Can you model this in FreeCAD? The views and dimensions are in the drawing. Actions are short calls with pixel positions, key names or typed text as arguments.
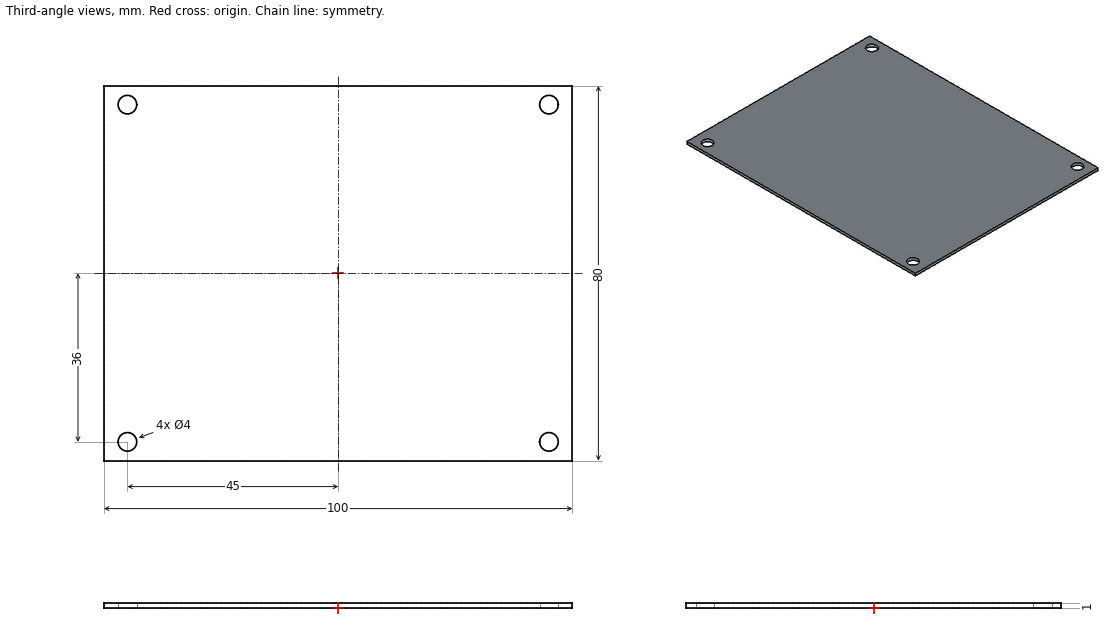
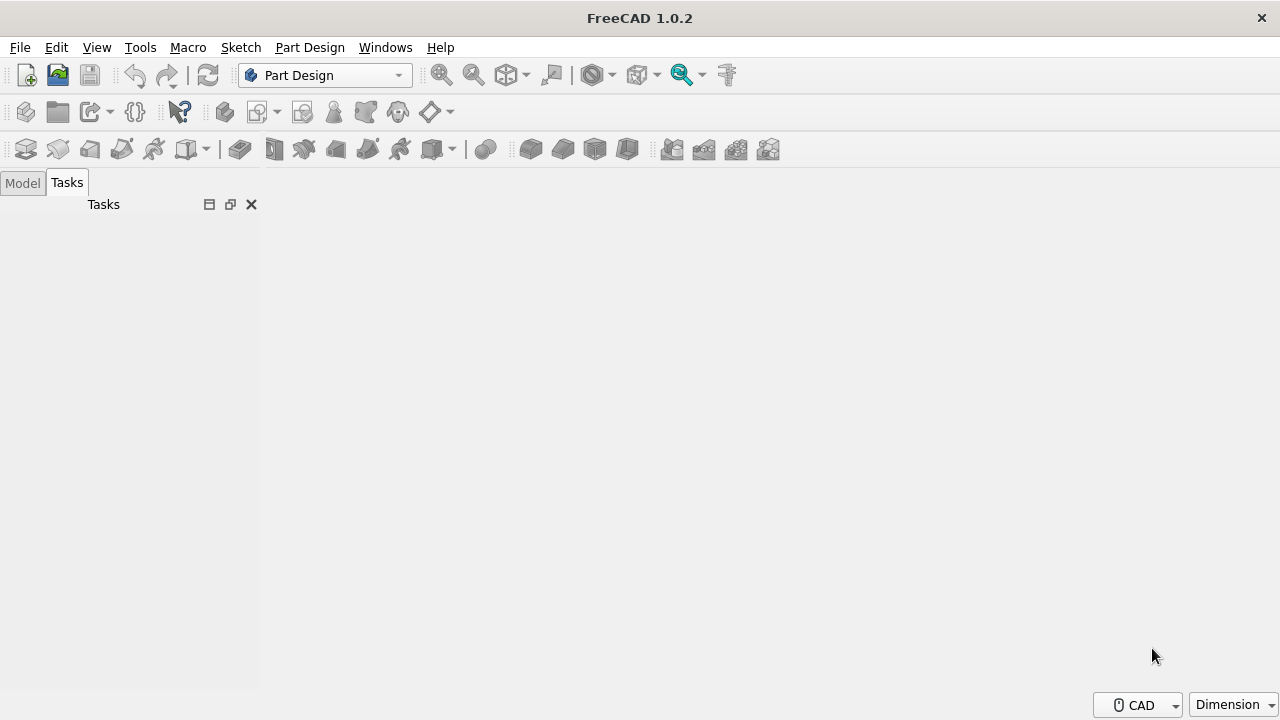
click(356, 76)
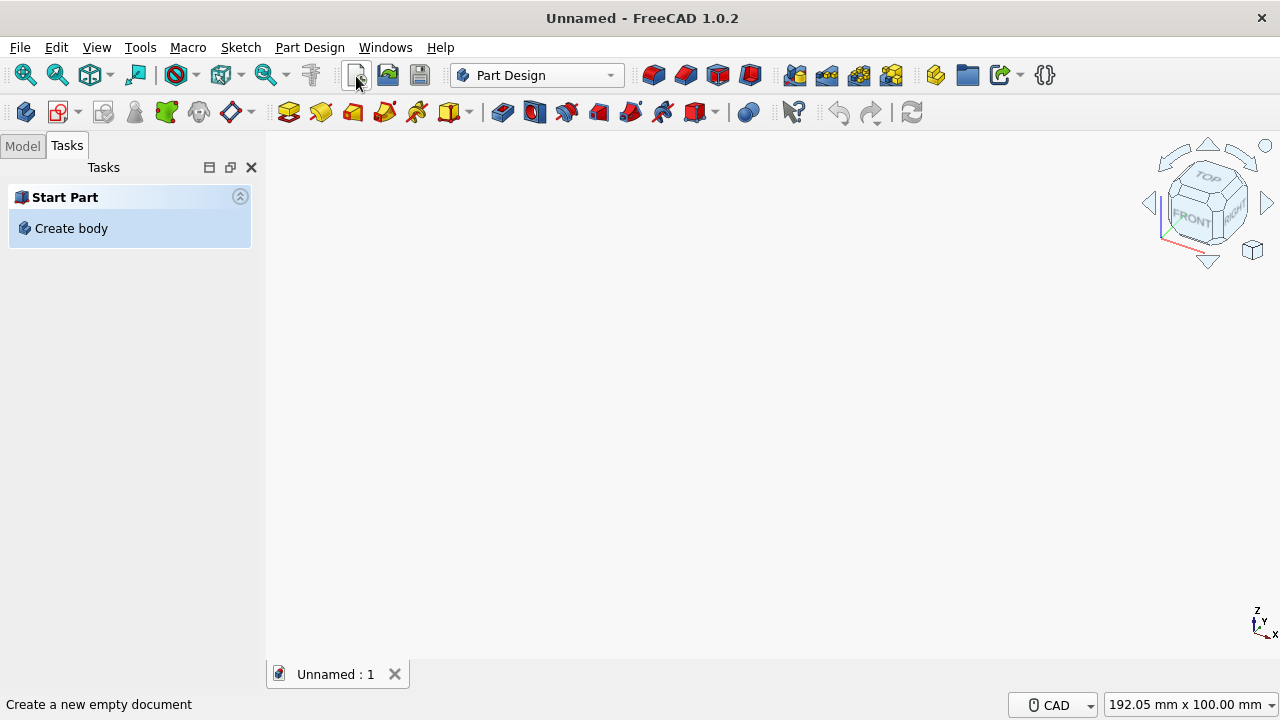
click(58, 112)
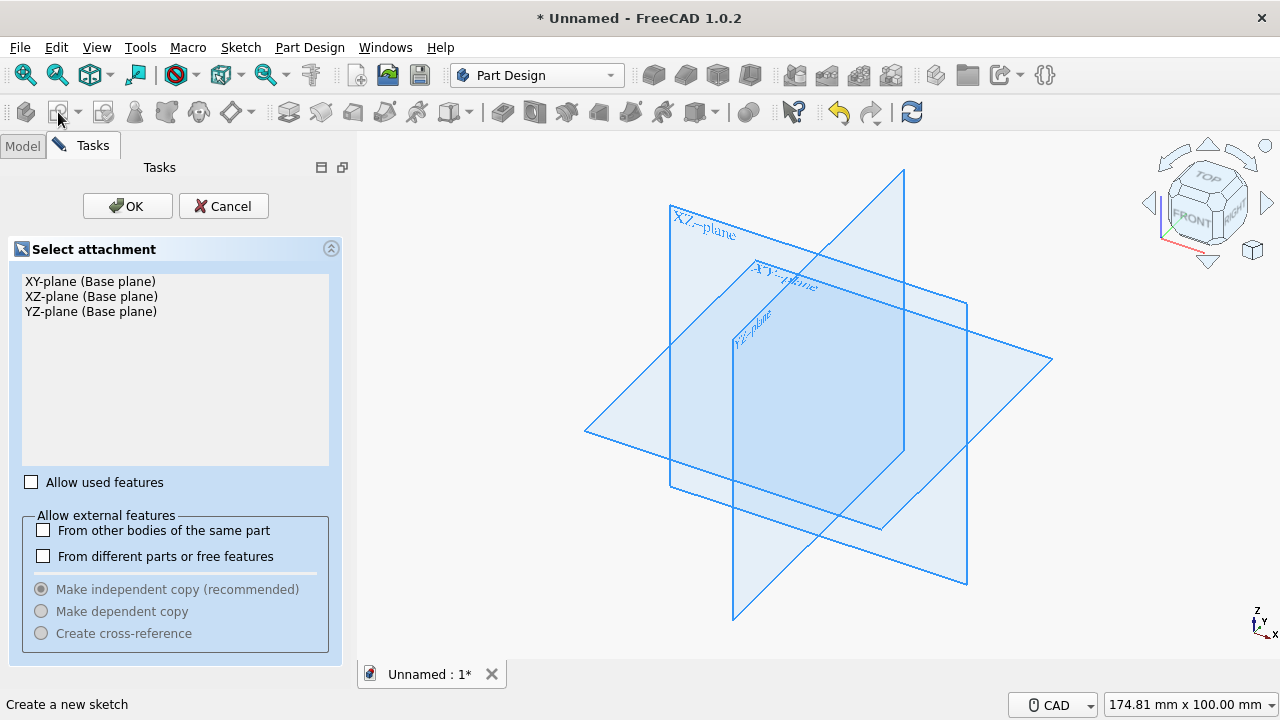
click(82, 282)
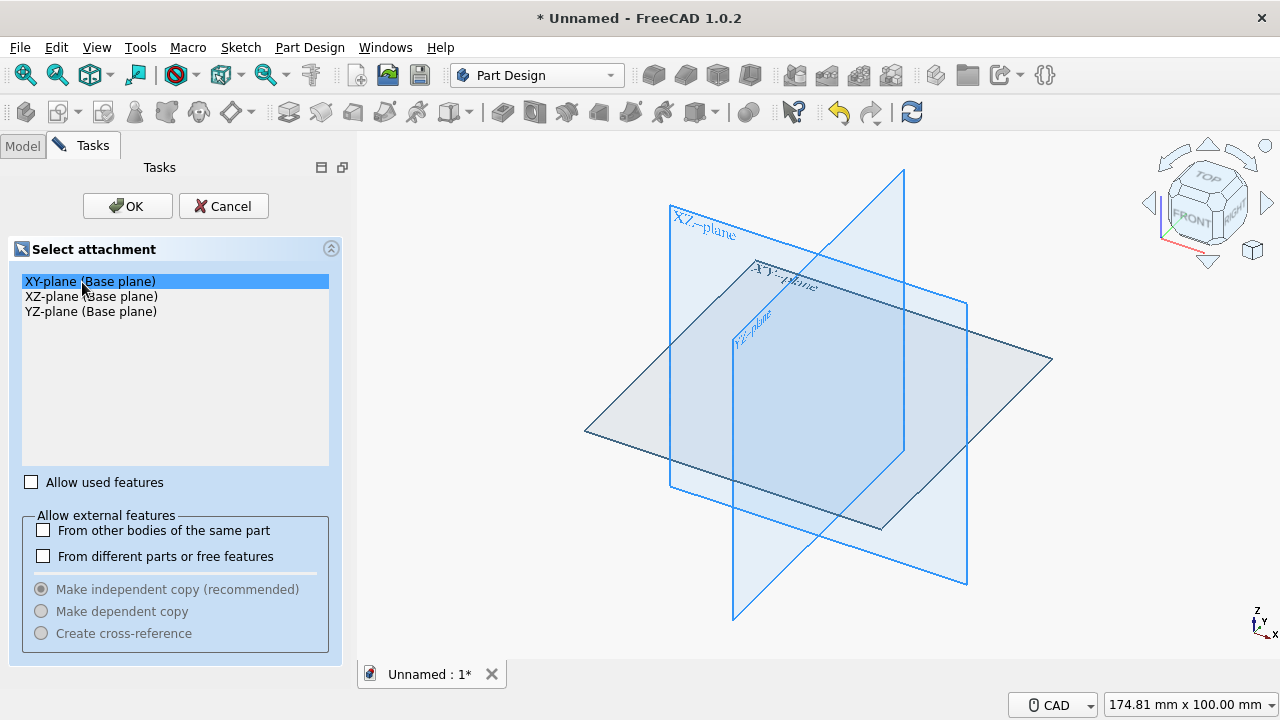
click(128, 206)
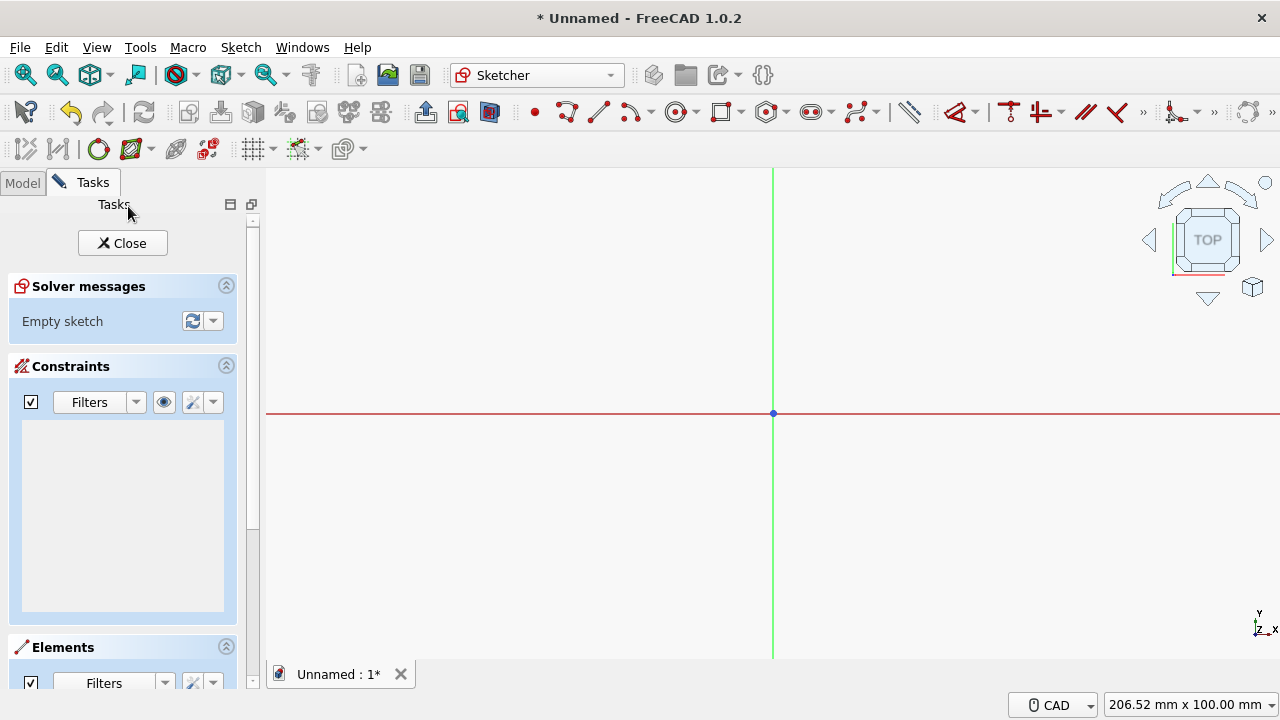
scroll(395, 413, down, 1)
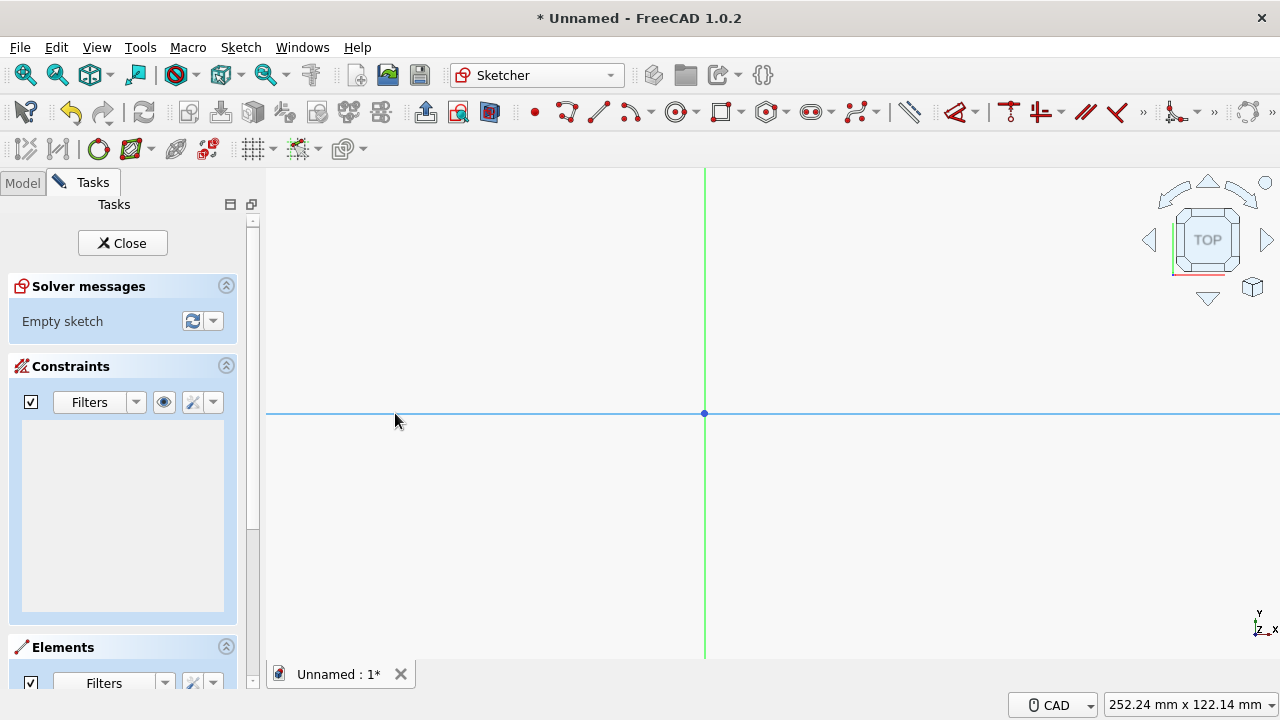
click(744, 112)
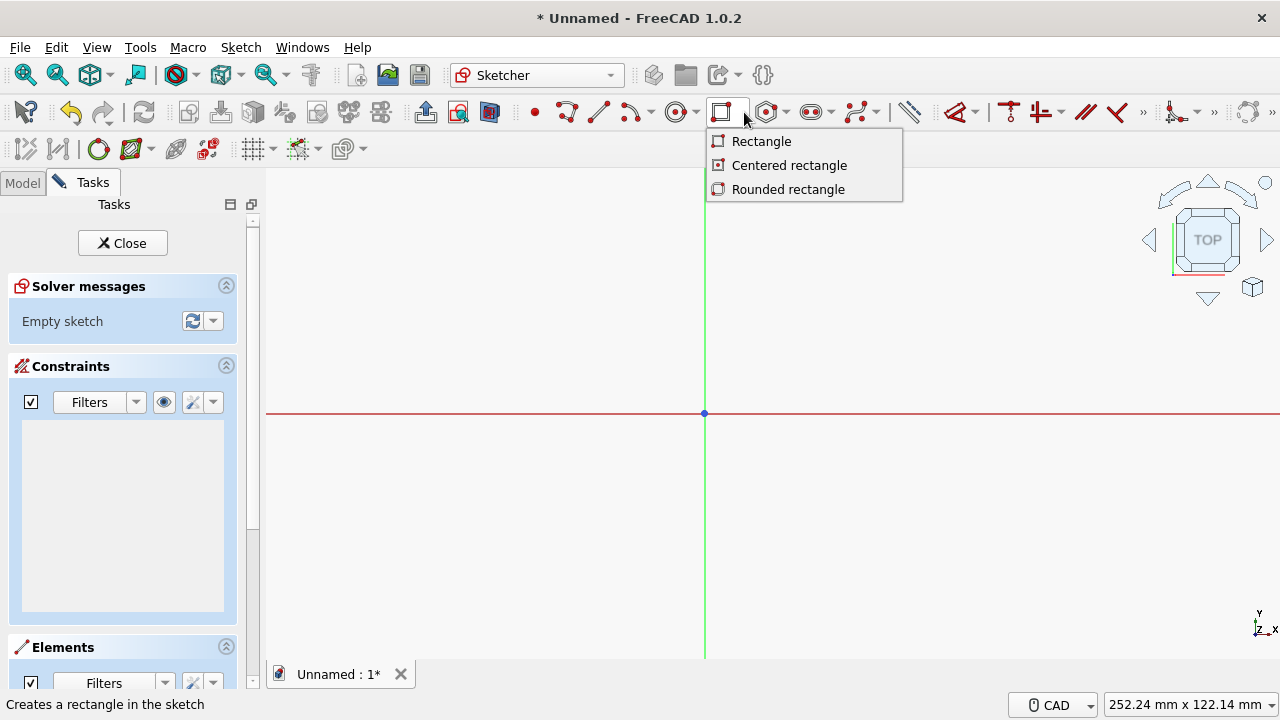
click(804, 165)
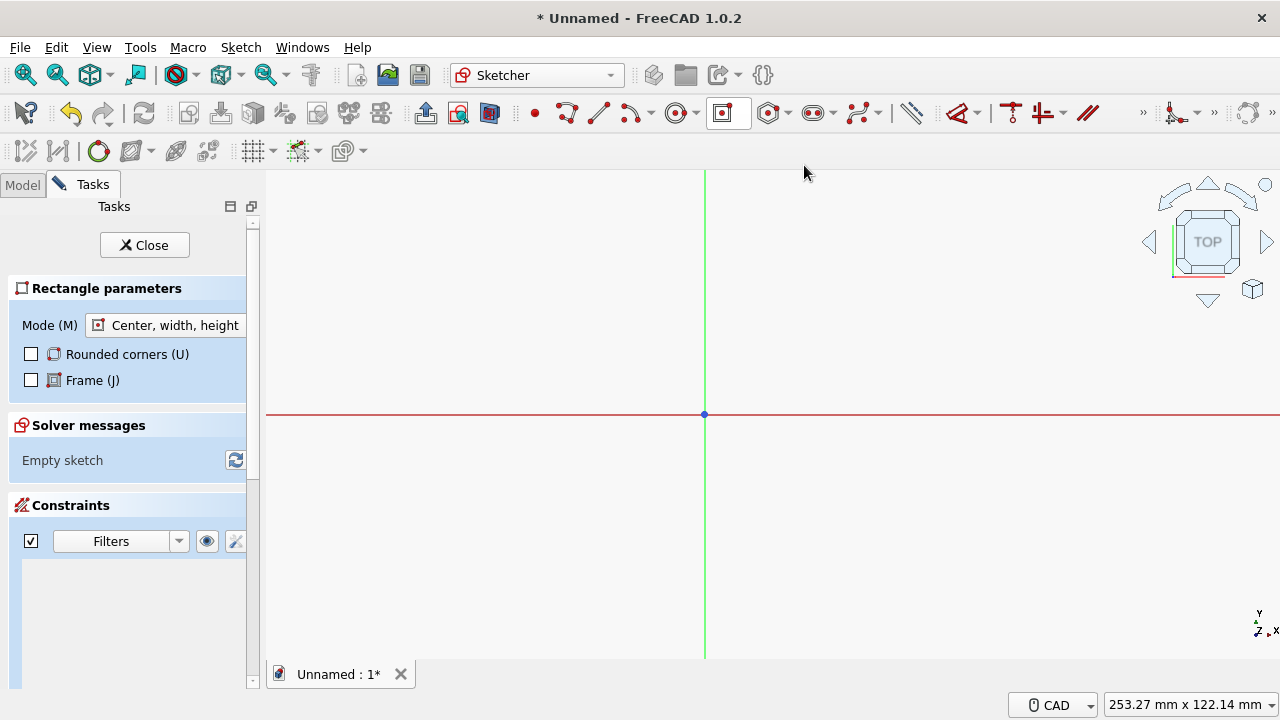
click(705, 414)
move(905, 254)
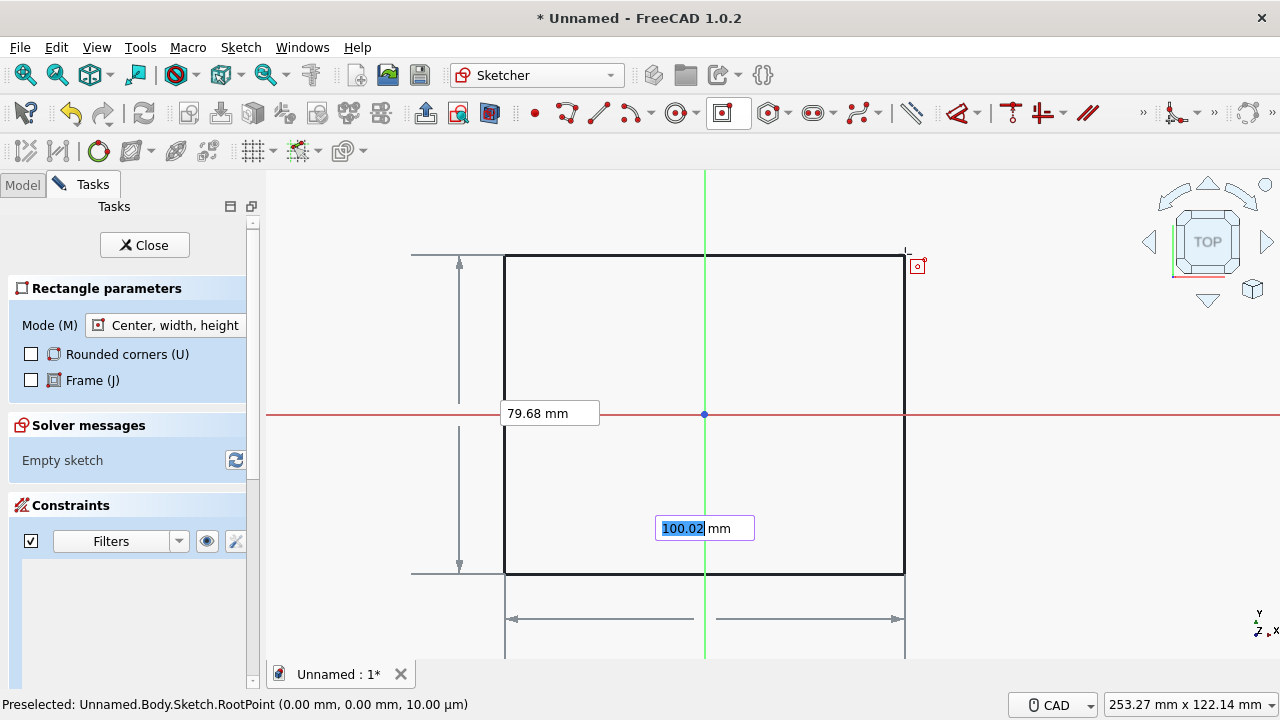
text(100)
key(Tab)
text(80)
key(Return)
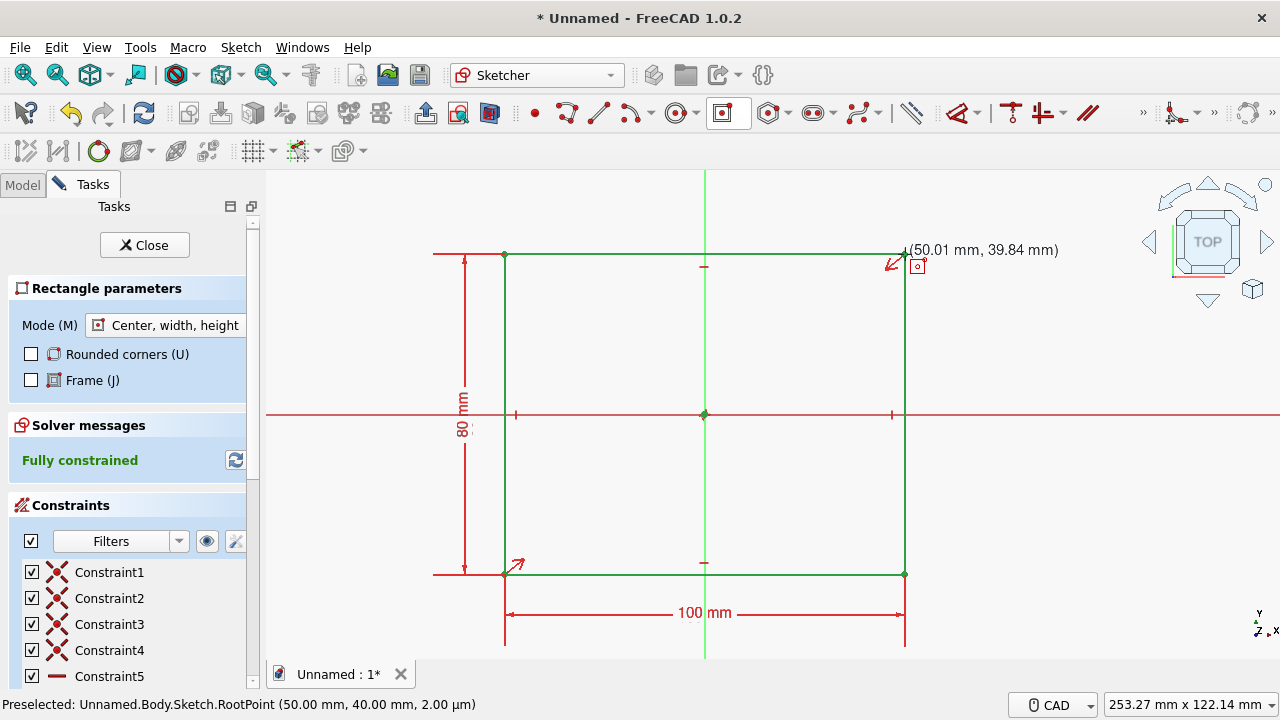
click(676, 114)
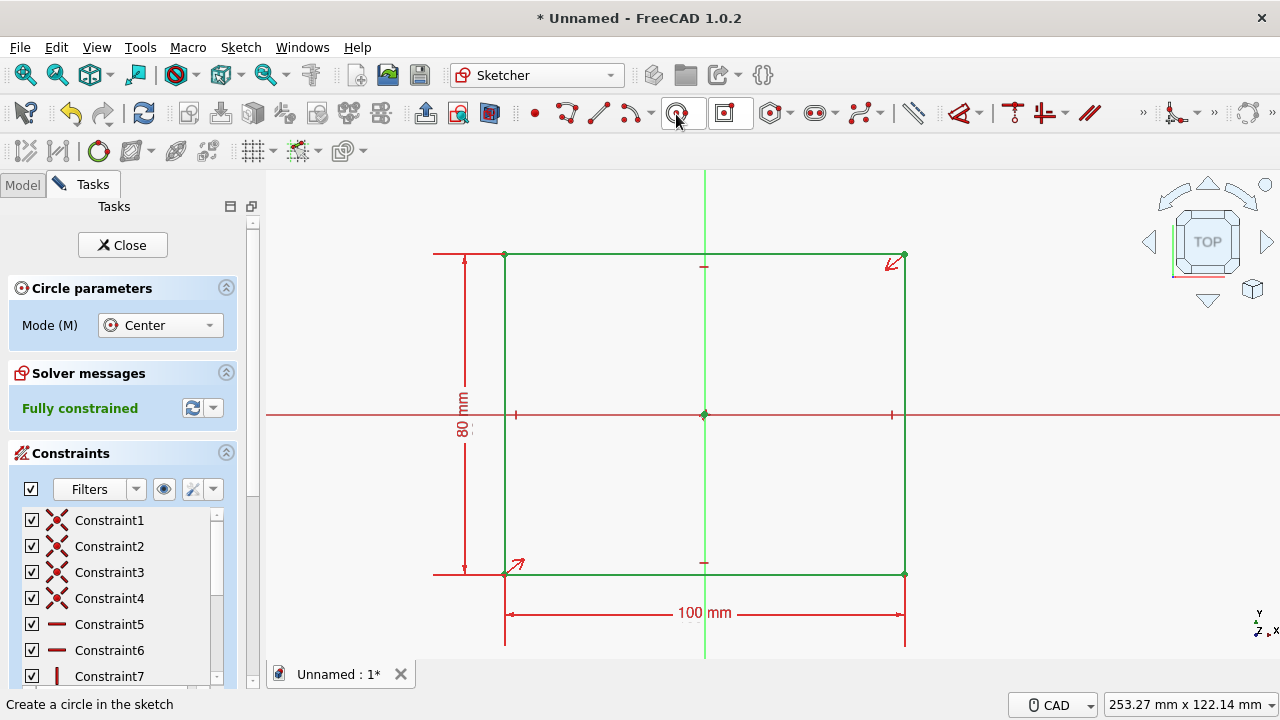
scroll(525, 559, up, 6)